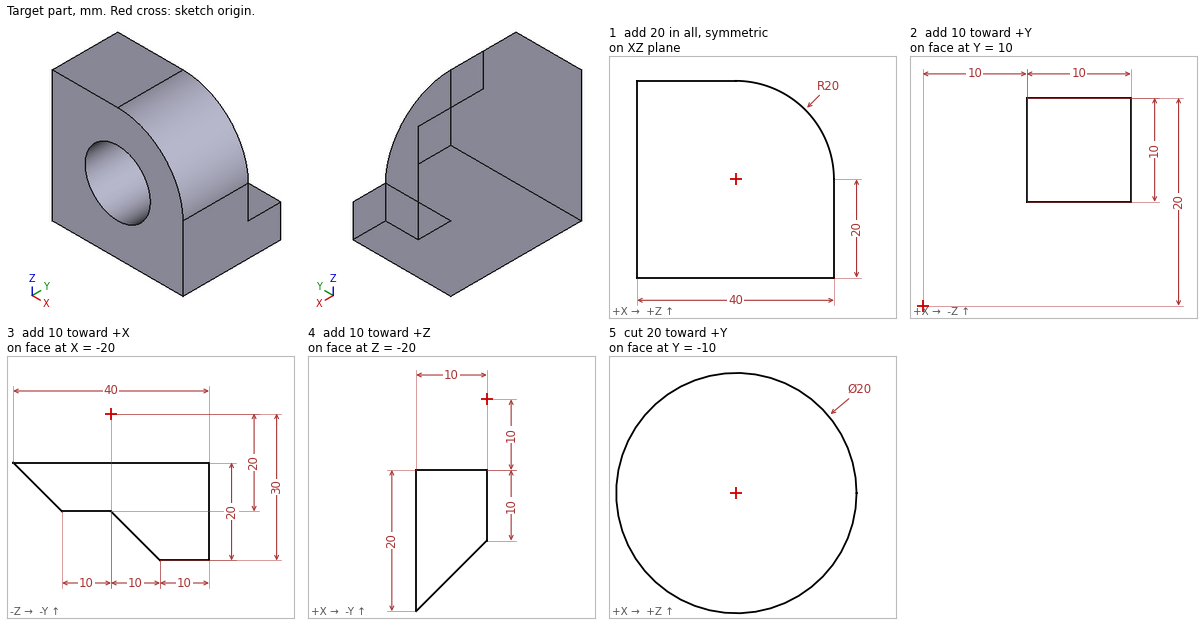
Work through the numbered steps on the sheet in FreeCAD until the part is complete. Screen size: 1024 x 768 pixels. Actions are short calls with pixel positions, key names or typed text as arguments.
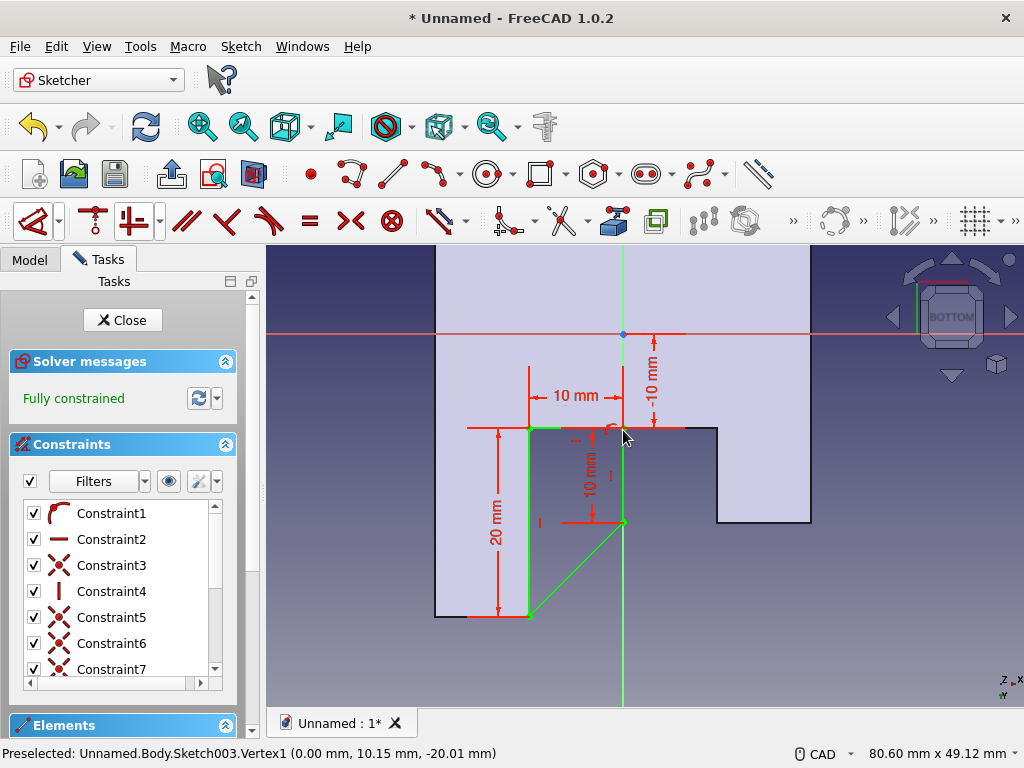
click(123, 320)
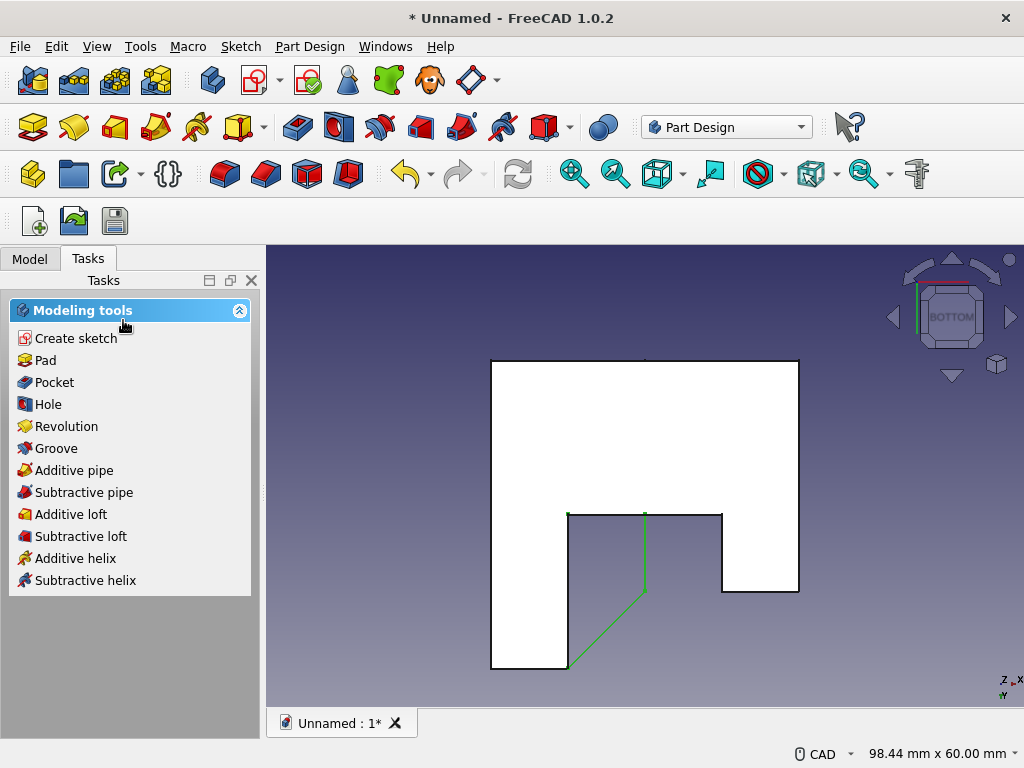
click(33, 128)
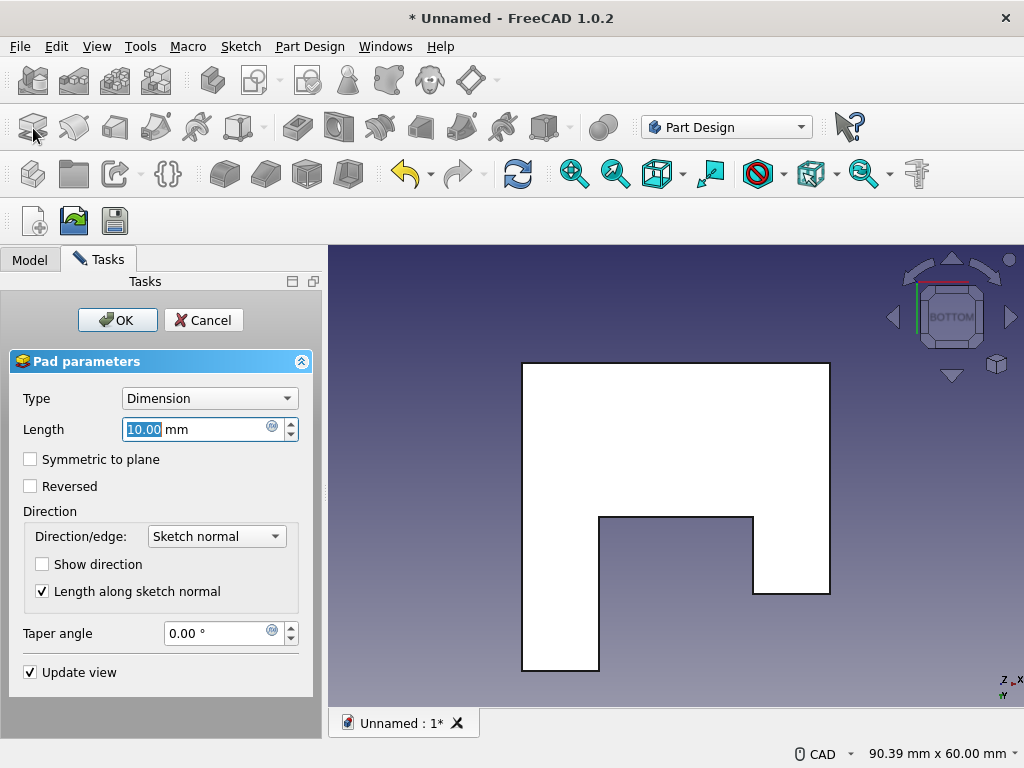
text(10)
key(Tab)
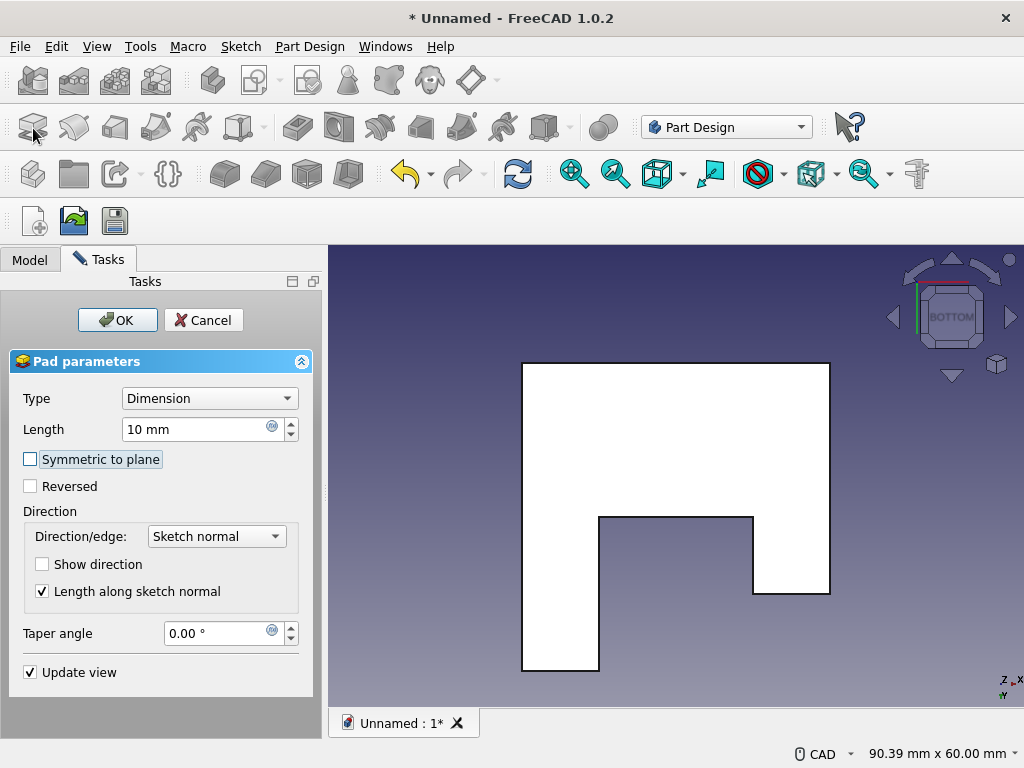
click(31, 486)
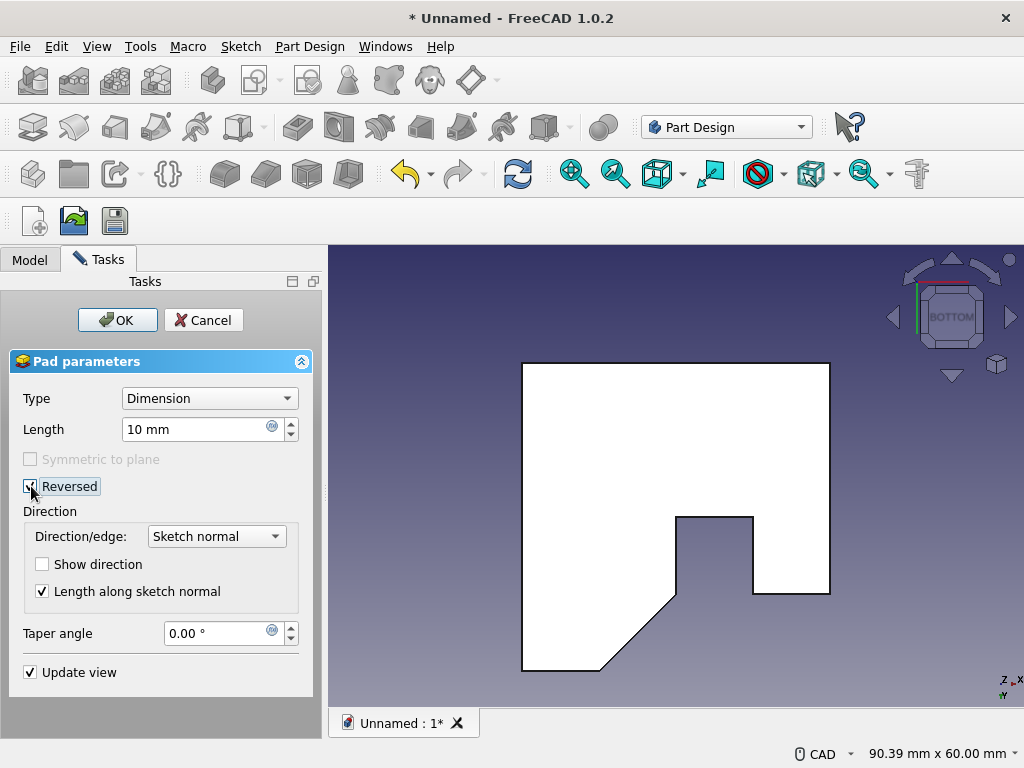
click(118, 320)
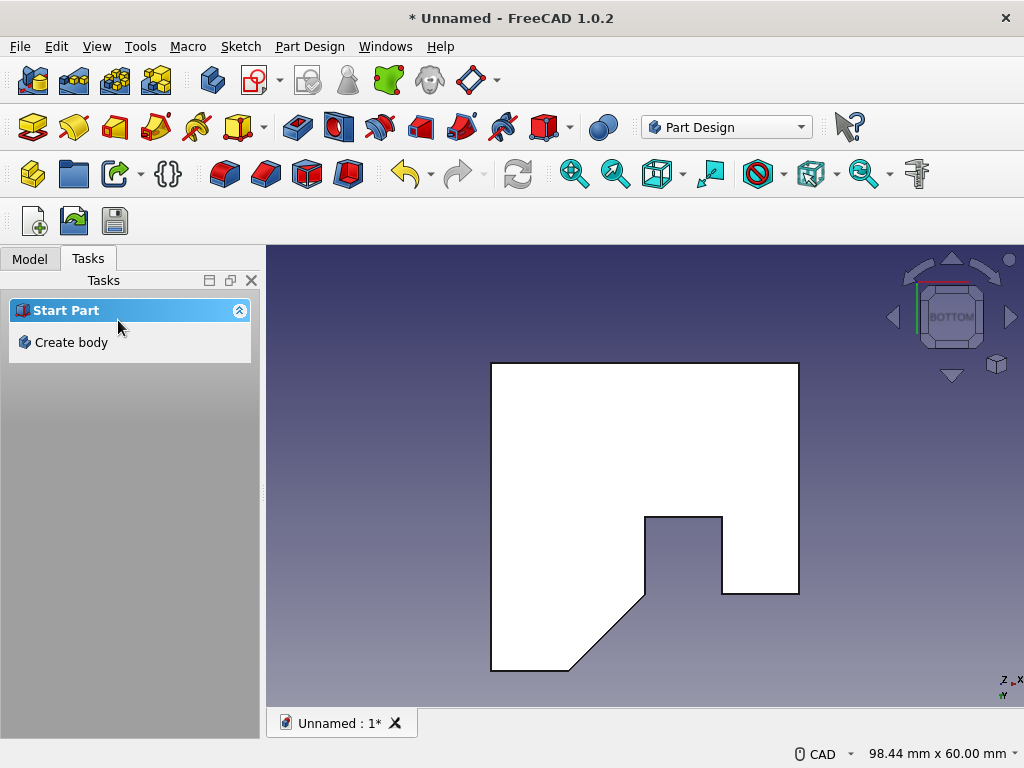
key(0)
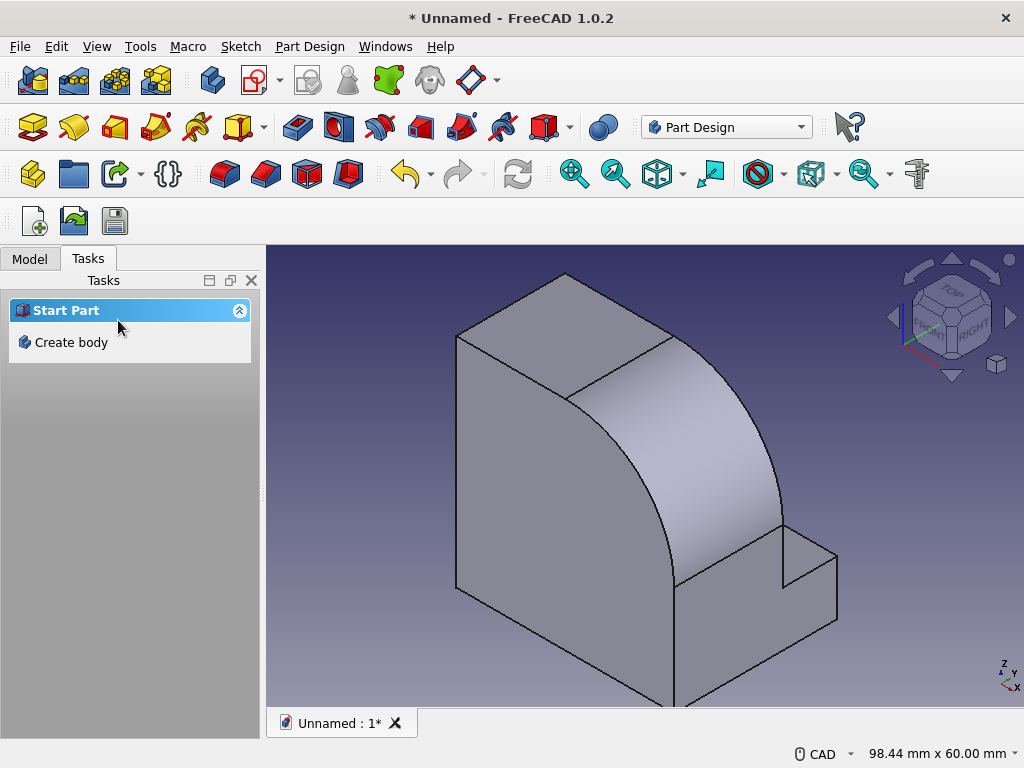
click(575, 174)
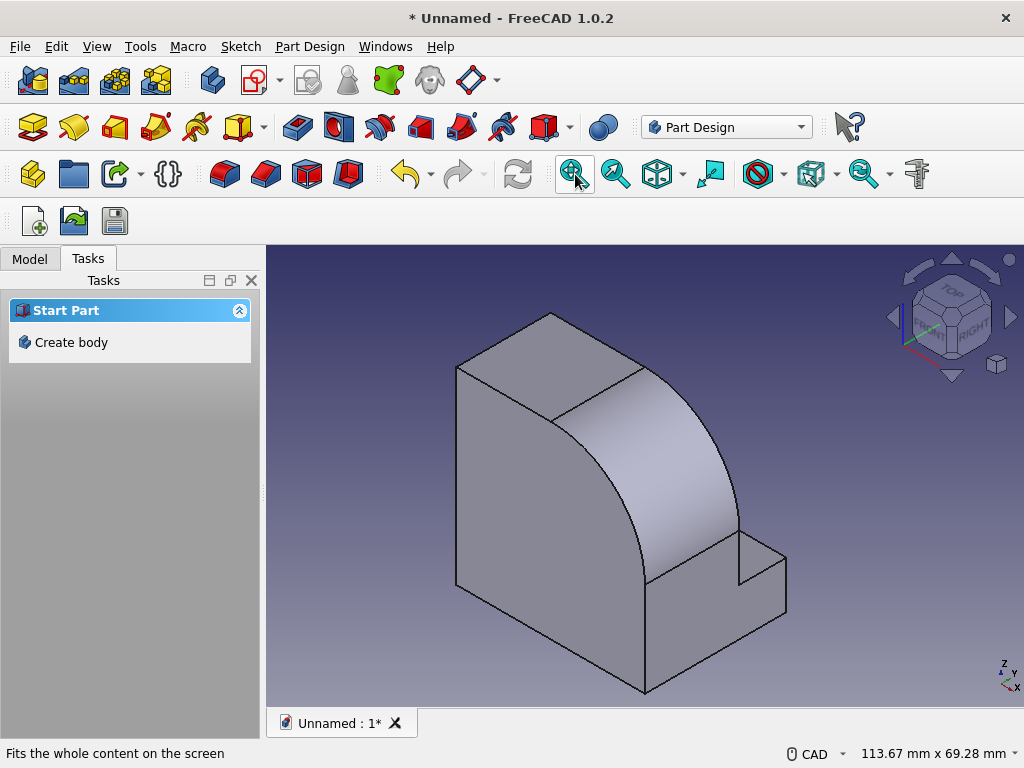
click(551, 529)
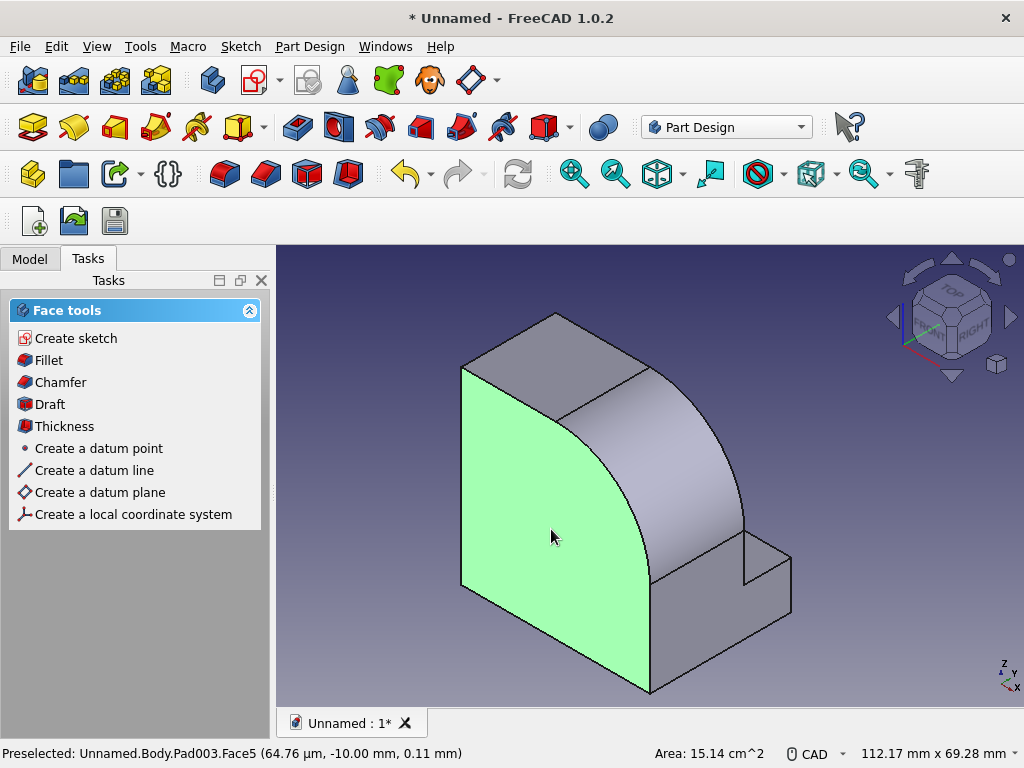
click(254, 80)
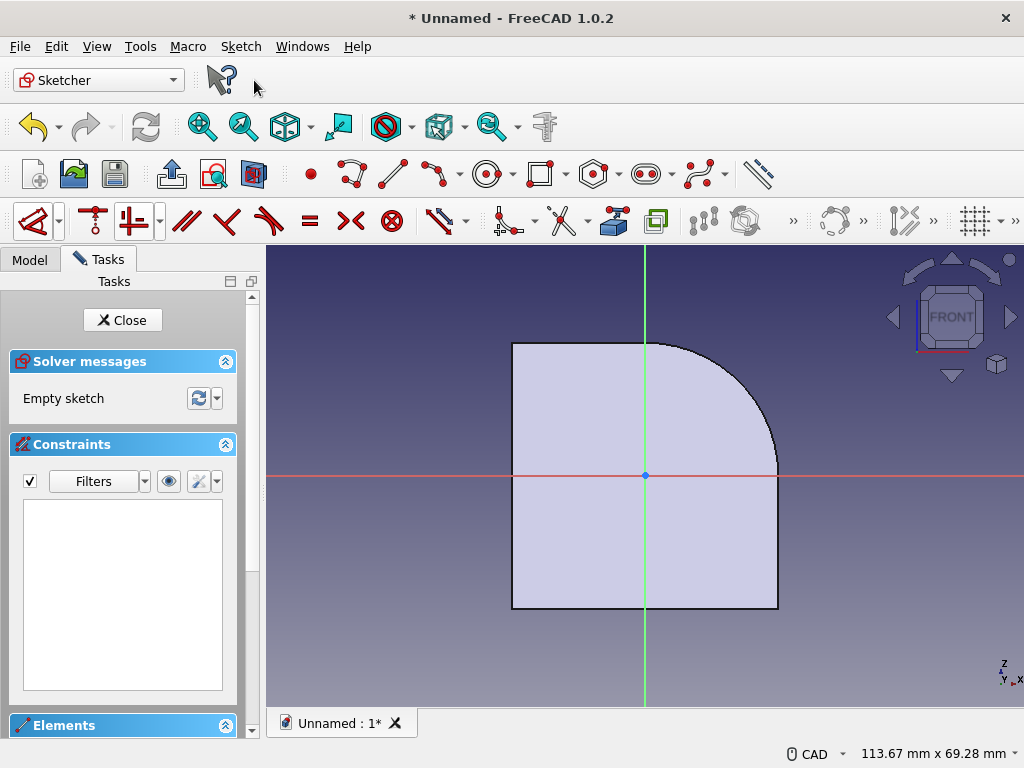
scroll(701, 476, up, 4)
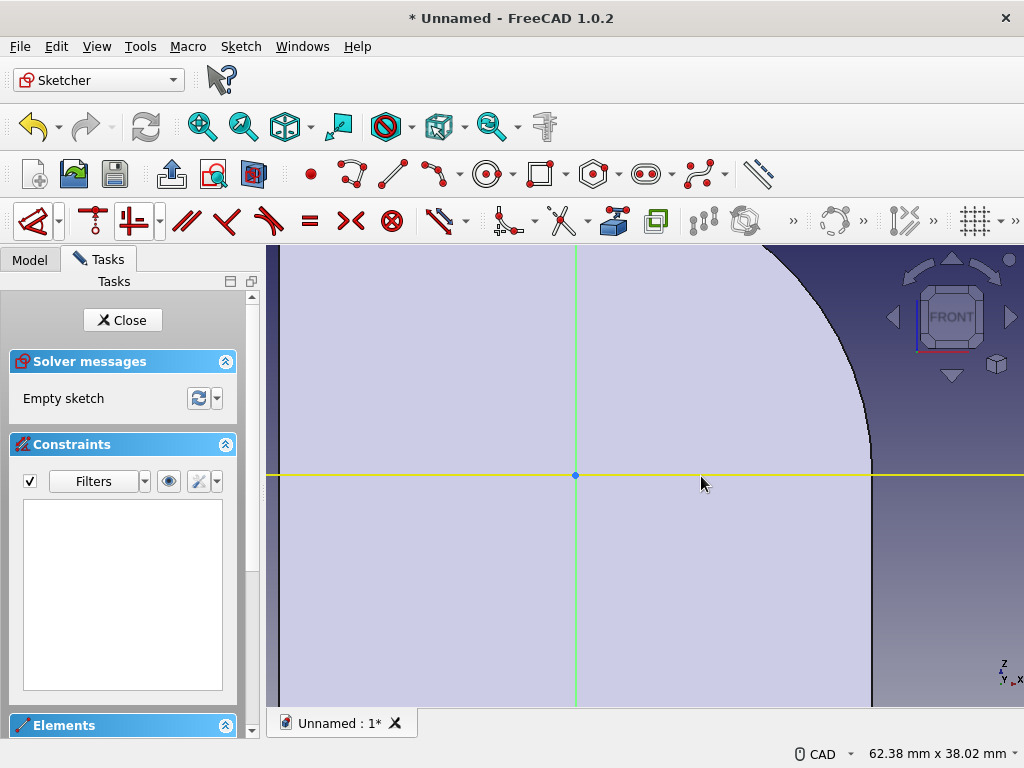
click(486, 174)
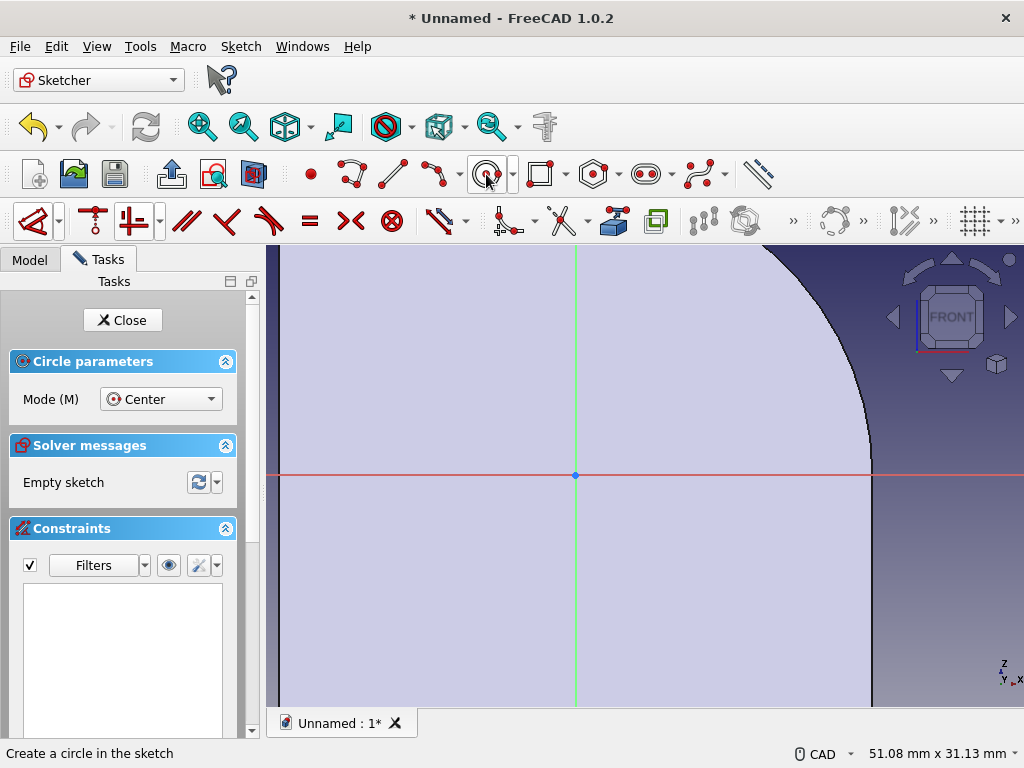
click(576, 475)
click(681, 370)
key(Escape)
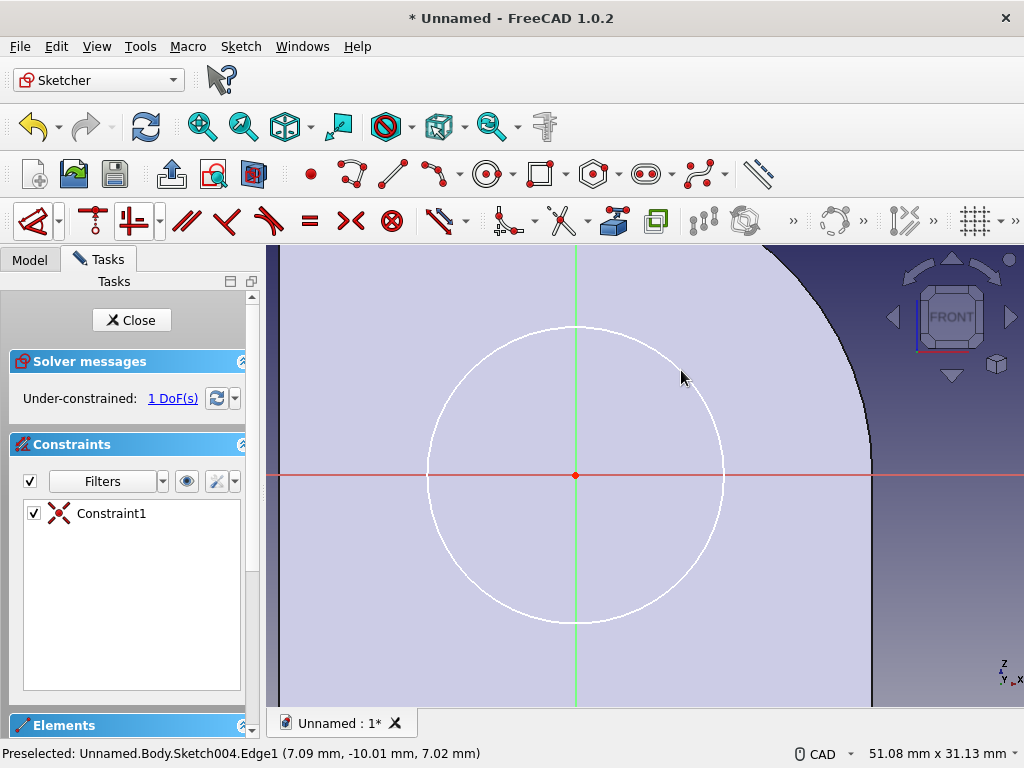
click(680, 370)